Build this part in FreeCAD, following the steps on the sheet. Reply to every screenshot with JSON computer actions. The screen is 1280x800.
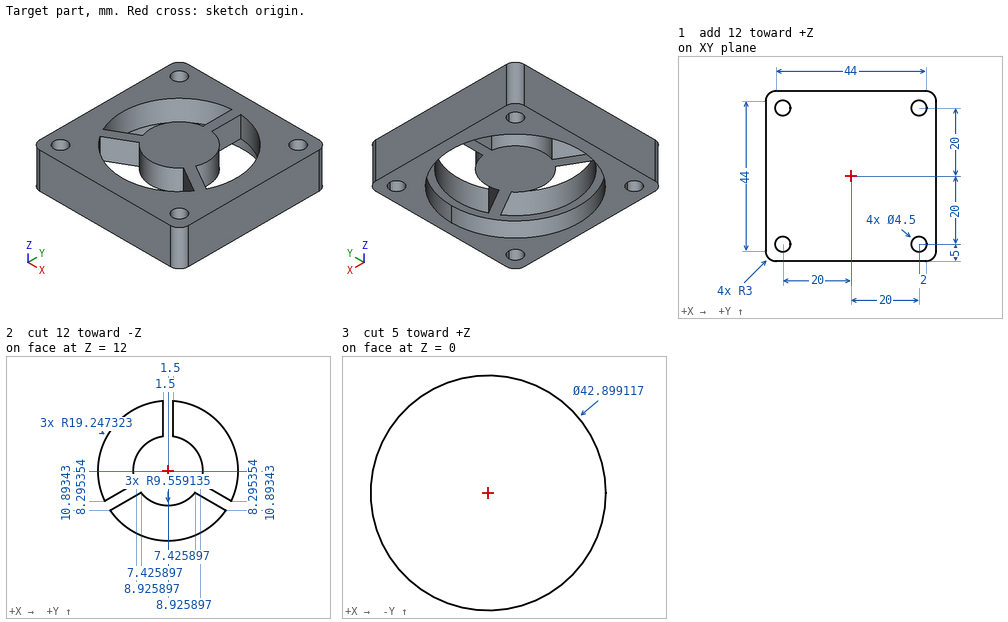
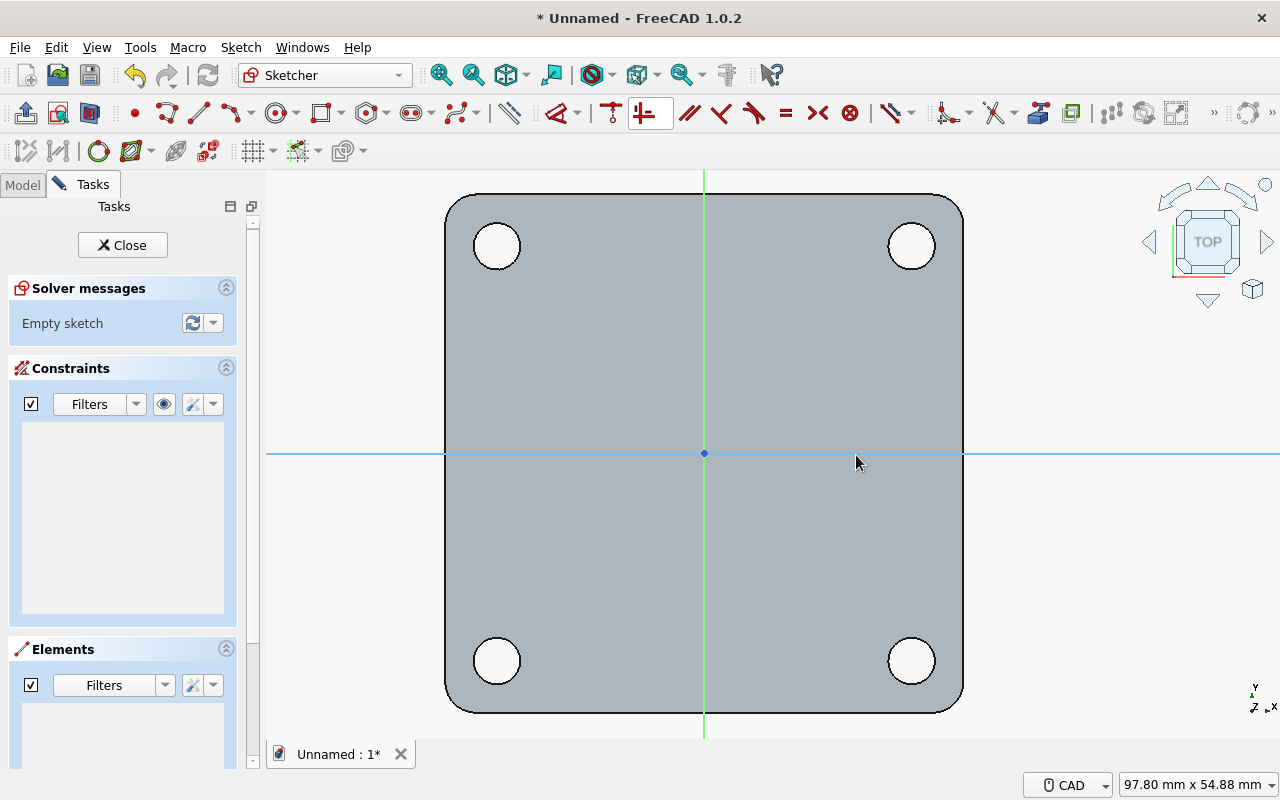
{"action": "left_click", "coordinate": [200, 114]}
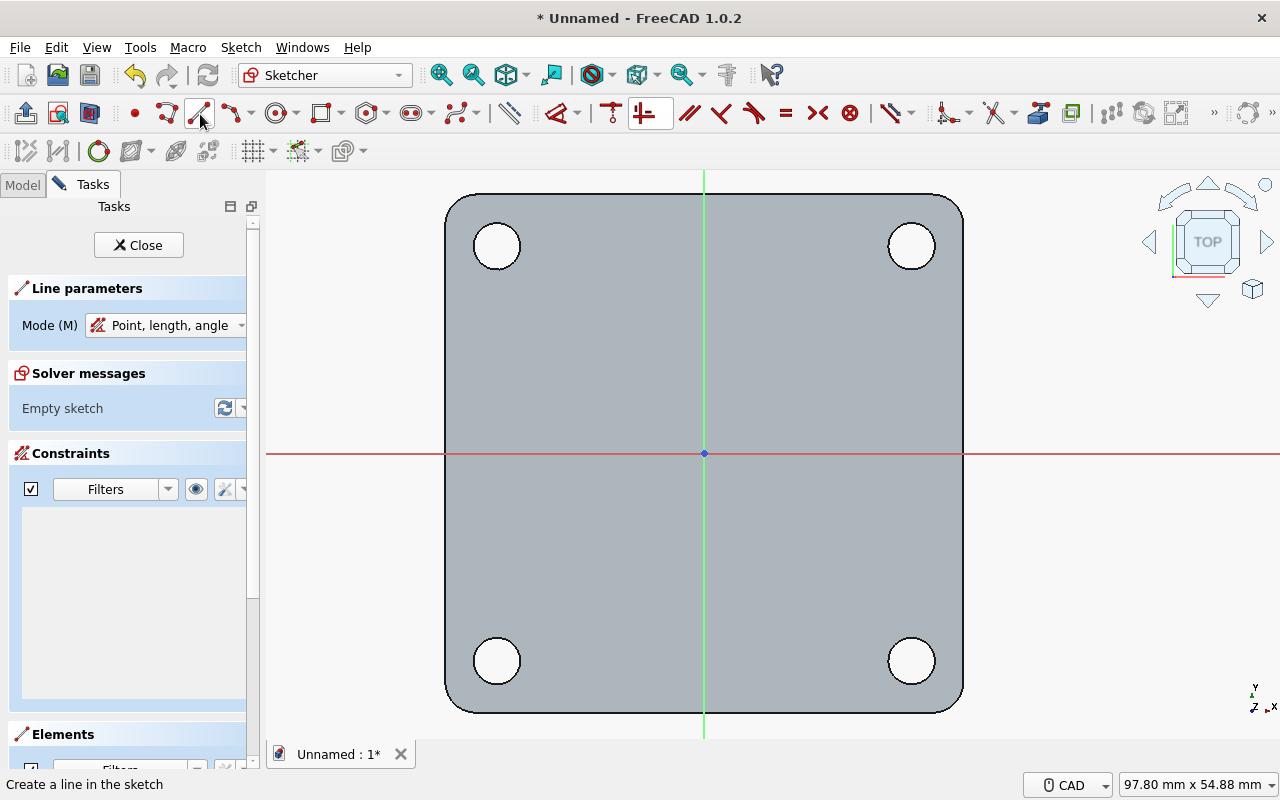
{"action": "left_click", "coordinate": [689, 356]}
{"action": "left_click", "coordinate": [689, 255]}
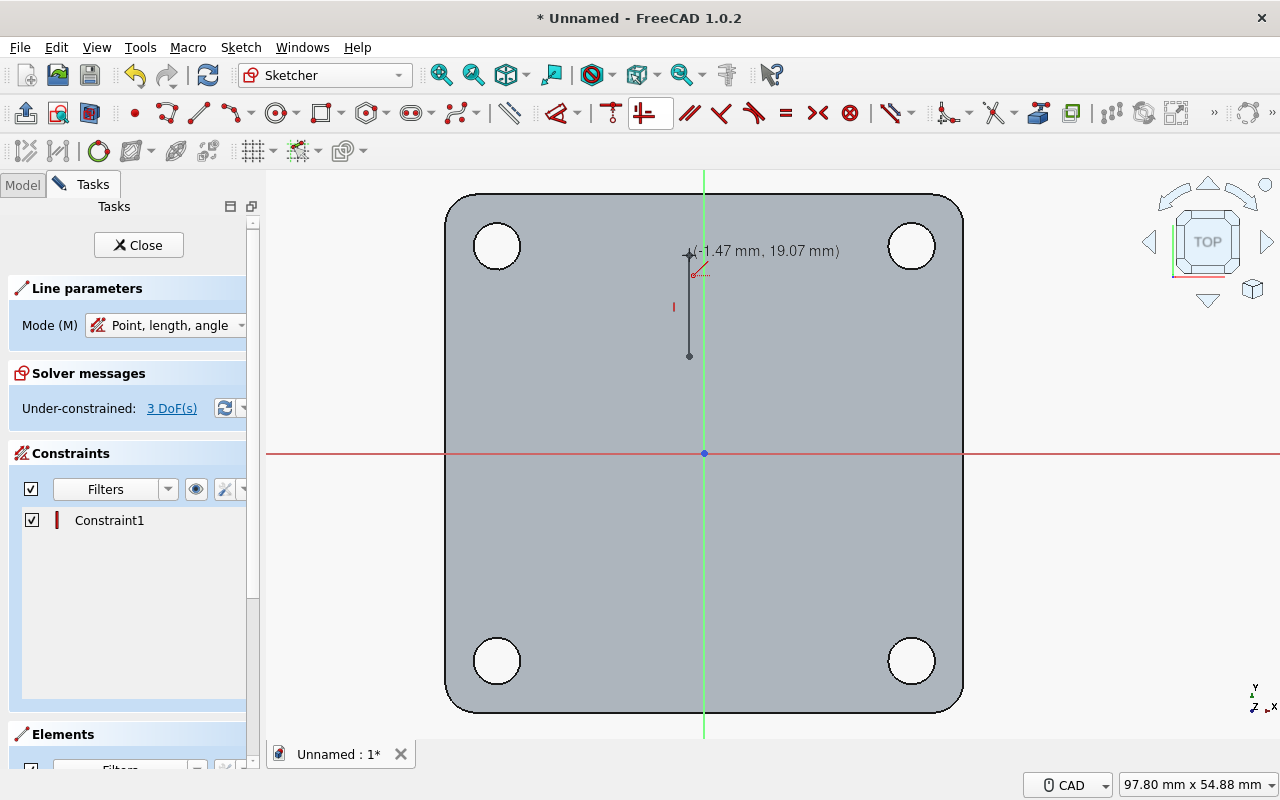
{"action": "left_click", "coordinate": [524, 540]}
{"action": "left_click", "coordinate": [612, 489]}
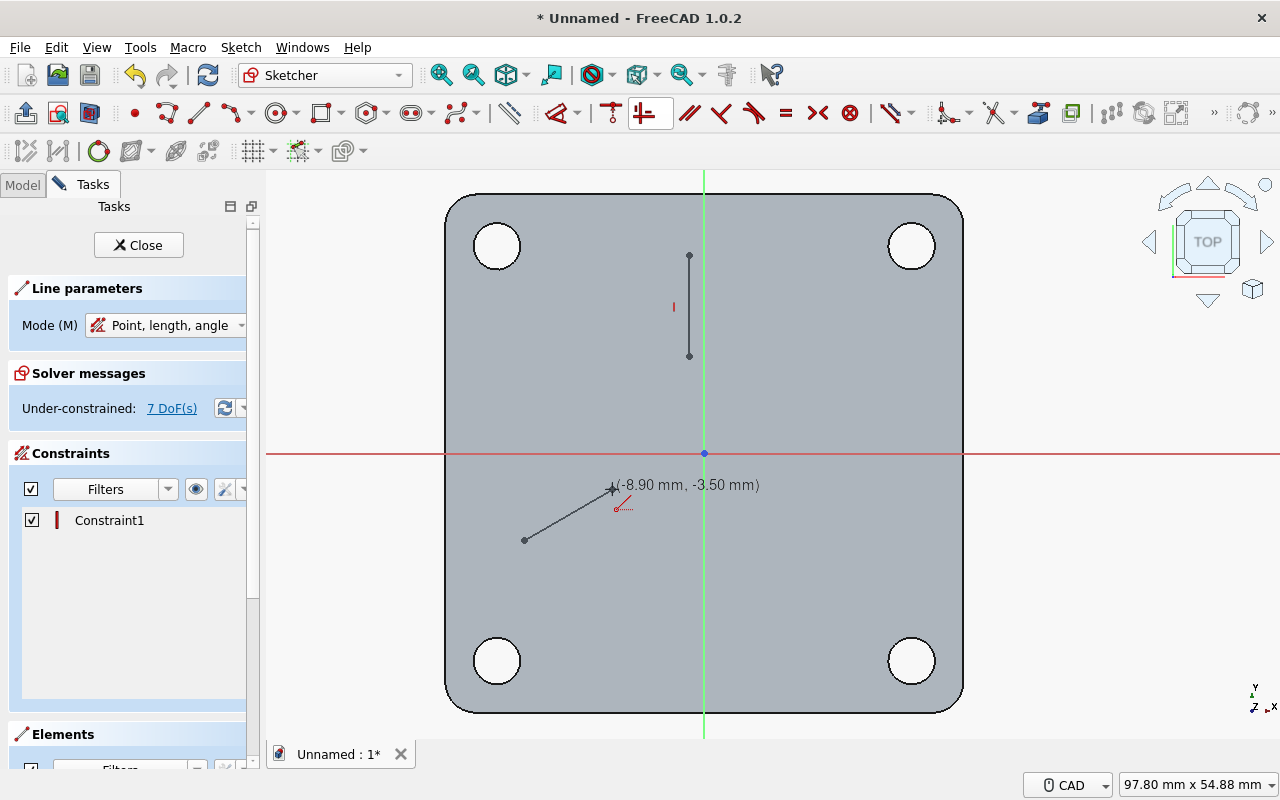
{"action": "left_click", "coordinate": [232, 114]}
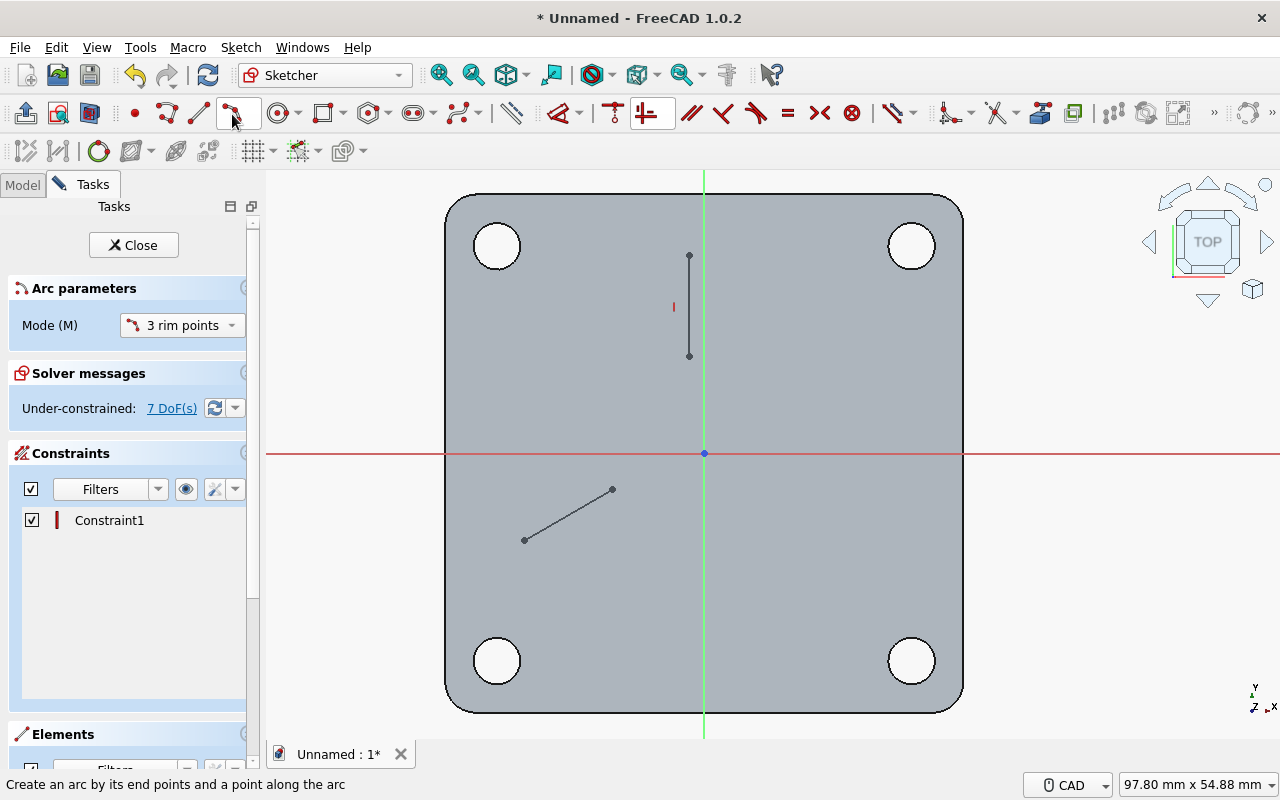
{"action": "left_click", "coordinate": [689, 256]}
{"action": "left_click", "coordinate": [524, 541]}
{"action": "left_click", "coordinate": [531, 354]}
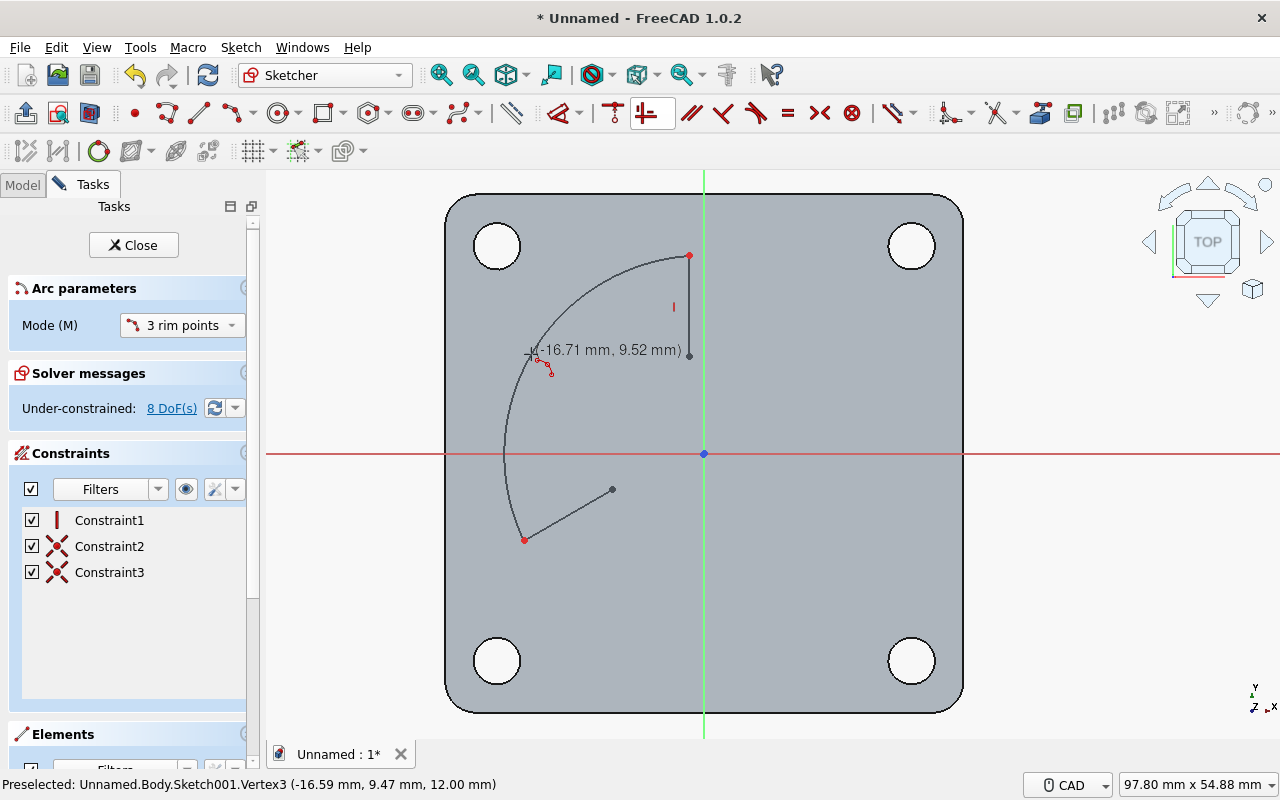
{"action": "left_click", "coordinate": [612, 490]}
{"action": "left_click", "coordinate": [689, 357]}
{"action": "left_click", "coordinate": [618, 404]}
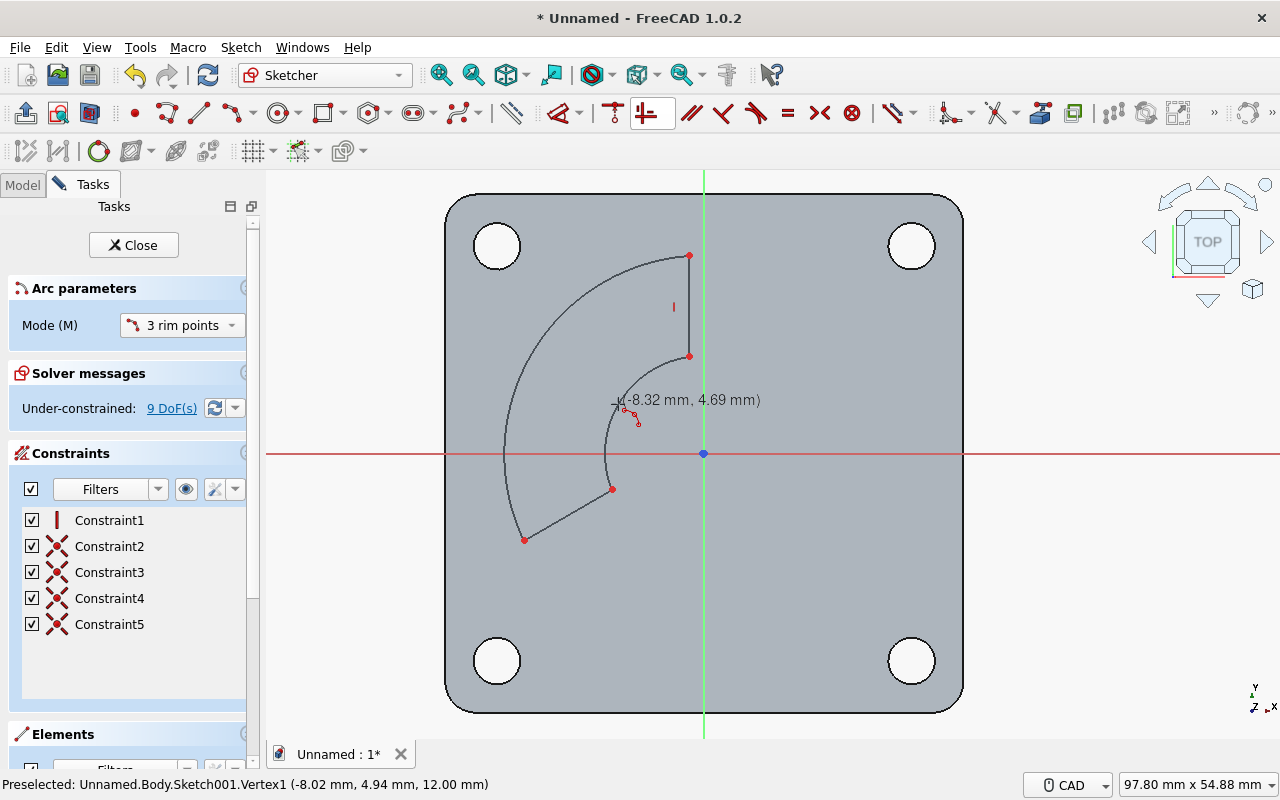
{"action": "left_click", "coordinate": [200, 114]}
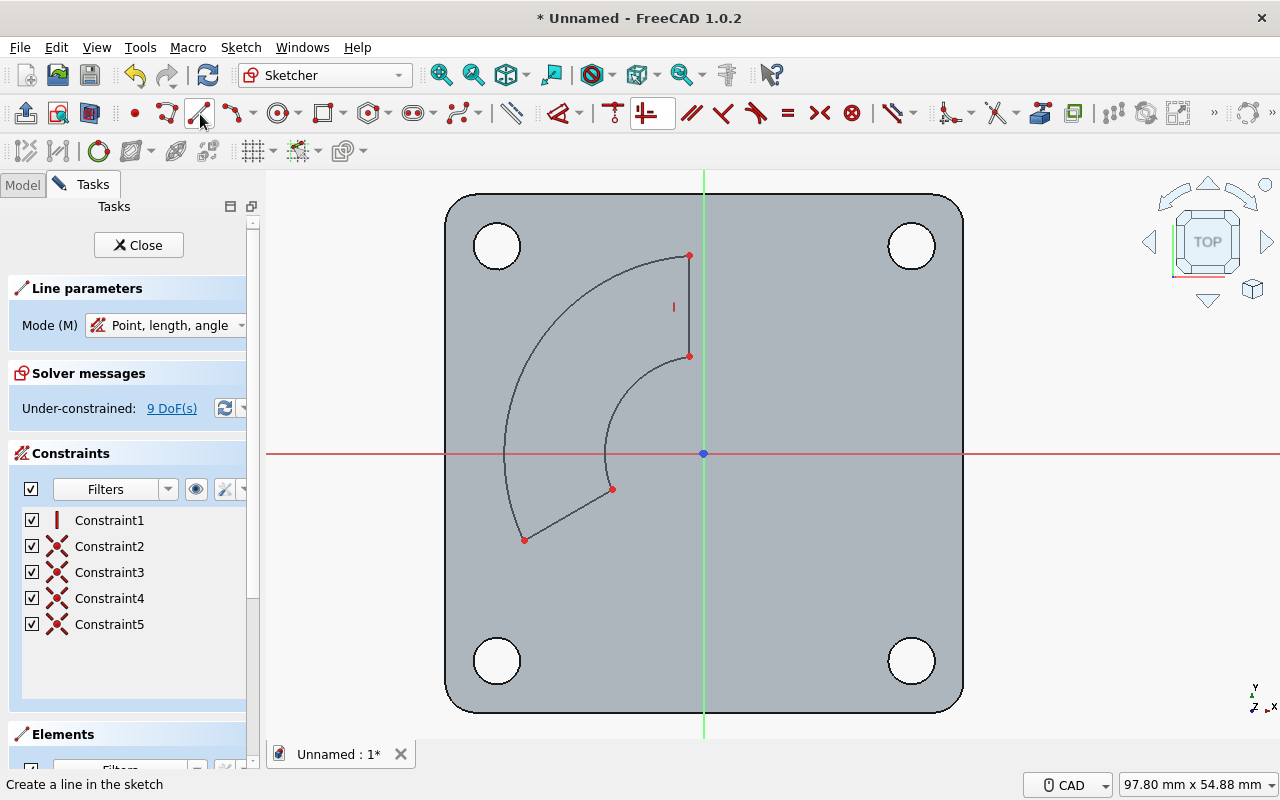
{"action": "left_click", "coordinate": [720, 255]}
{"action": "left_click", "coordinate": [720, 356]}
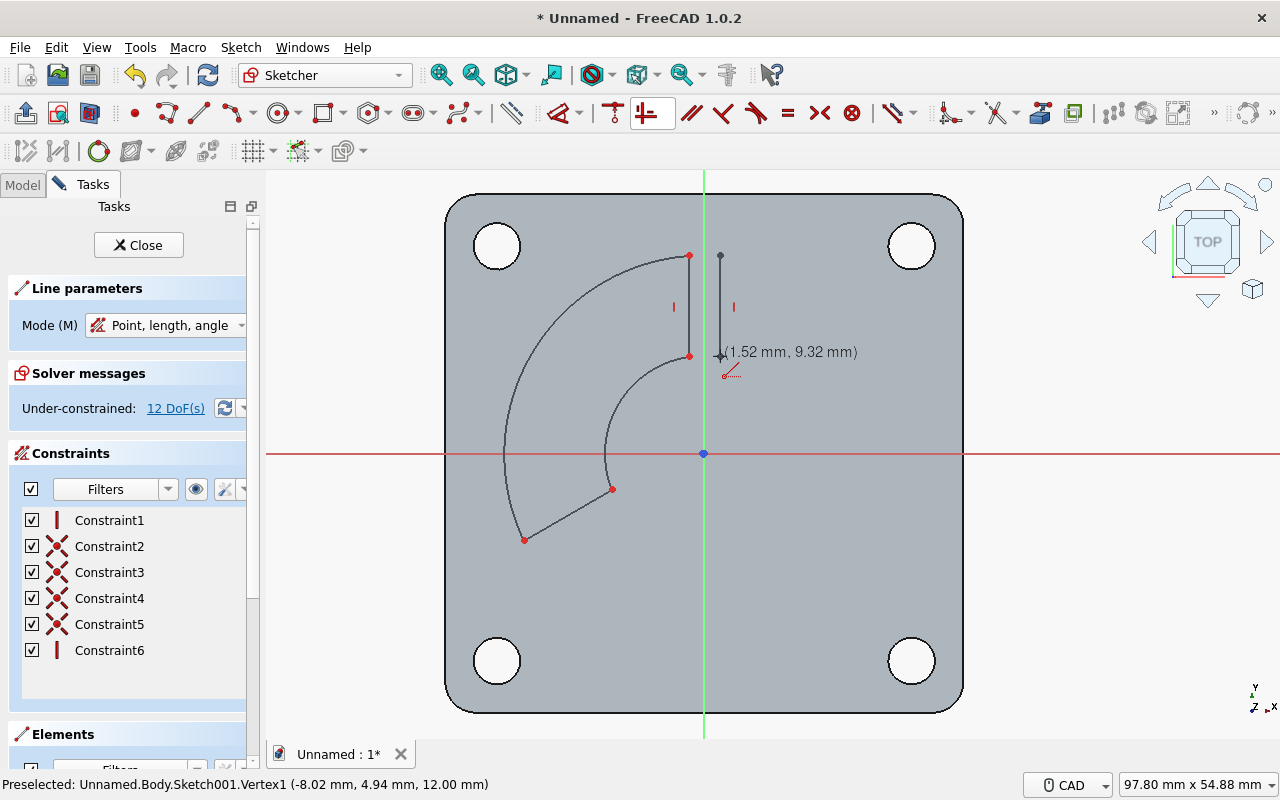
{"action": "left_click", "coordinate": [797, 489]}
{"action": "left_click", "coordinate": [884, 540]}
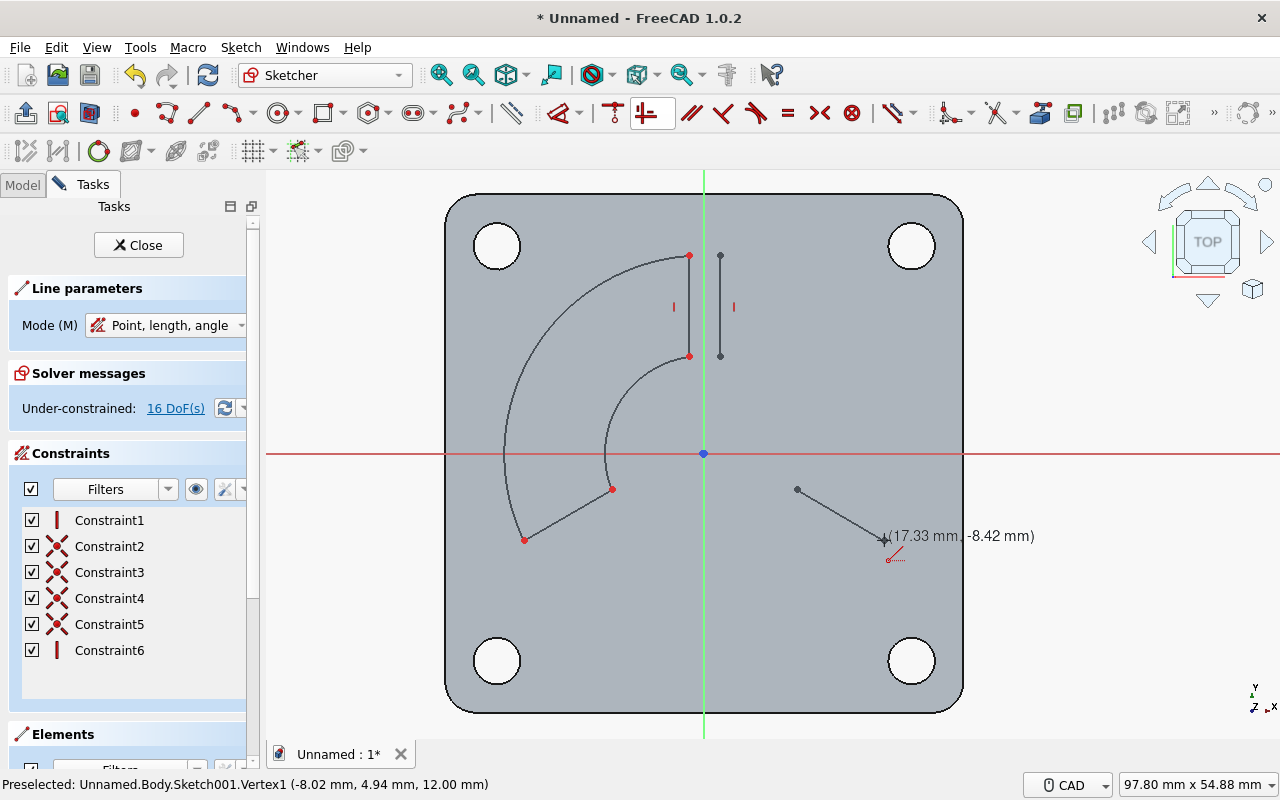
{"action": "left_click", "coordinate": [232, 114]}